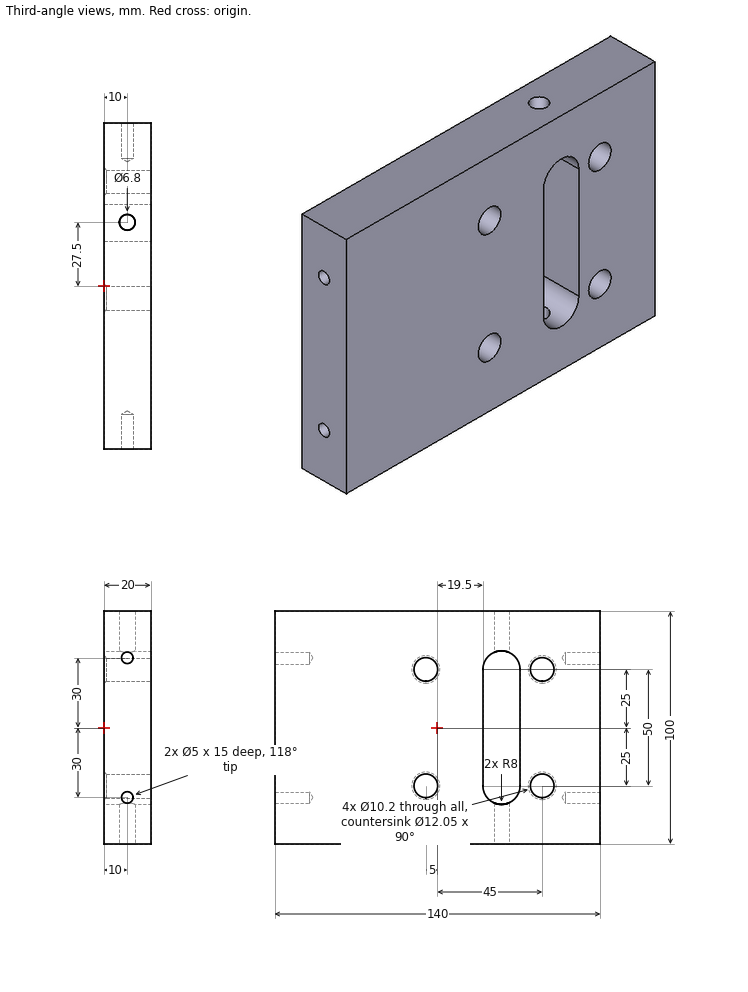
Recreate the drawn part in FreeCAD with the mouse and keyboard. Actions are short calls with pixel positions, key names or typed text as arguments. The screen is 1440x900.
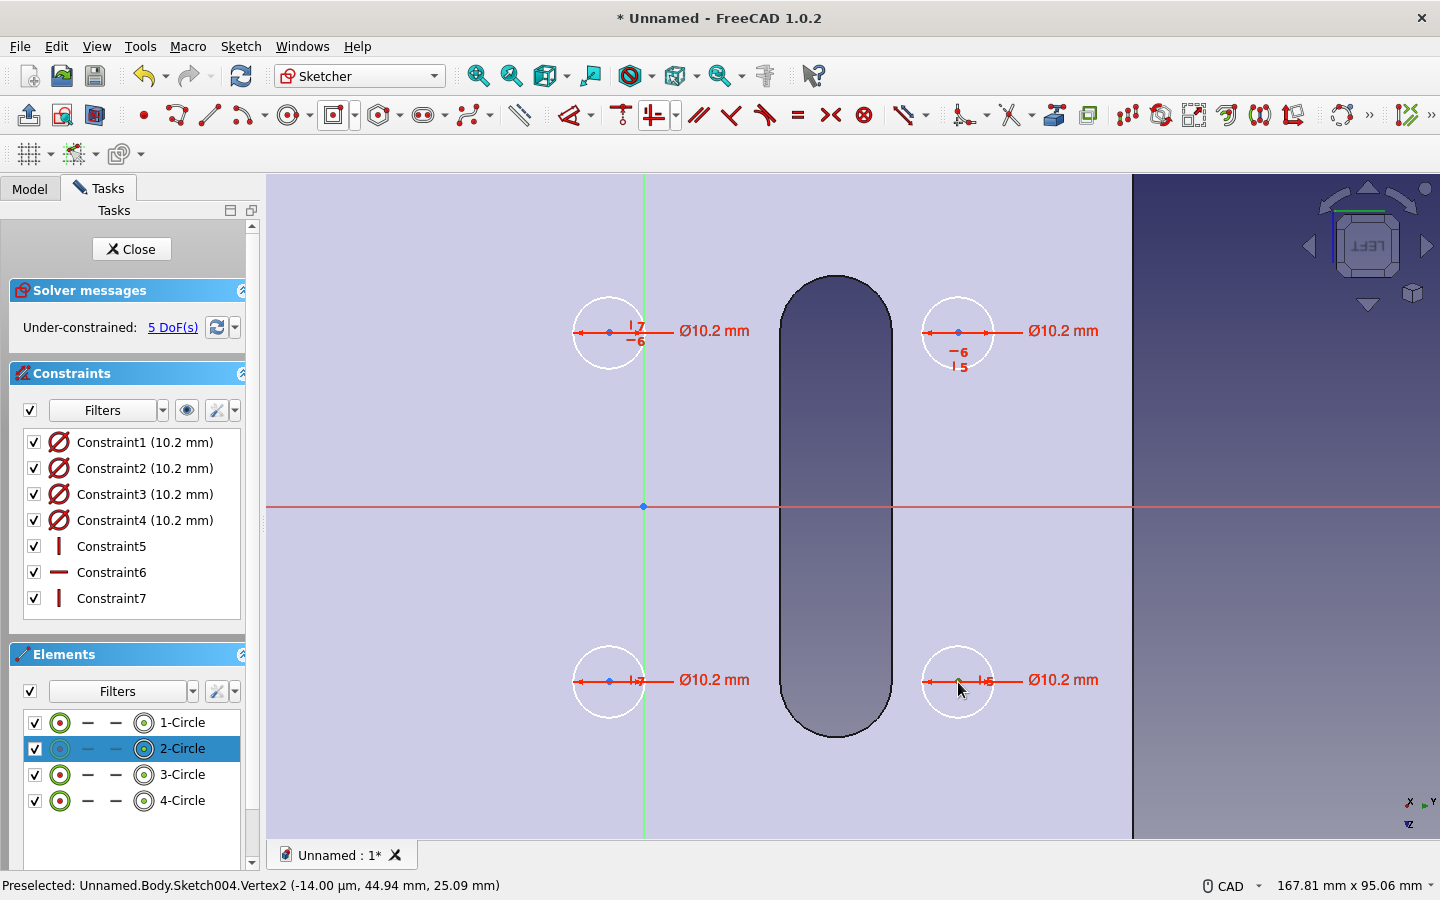
click(609, 682)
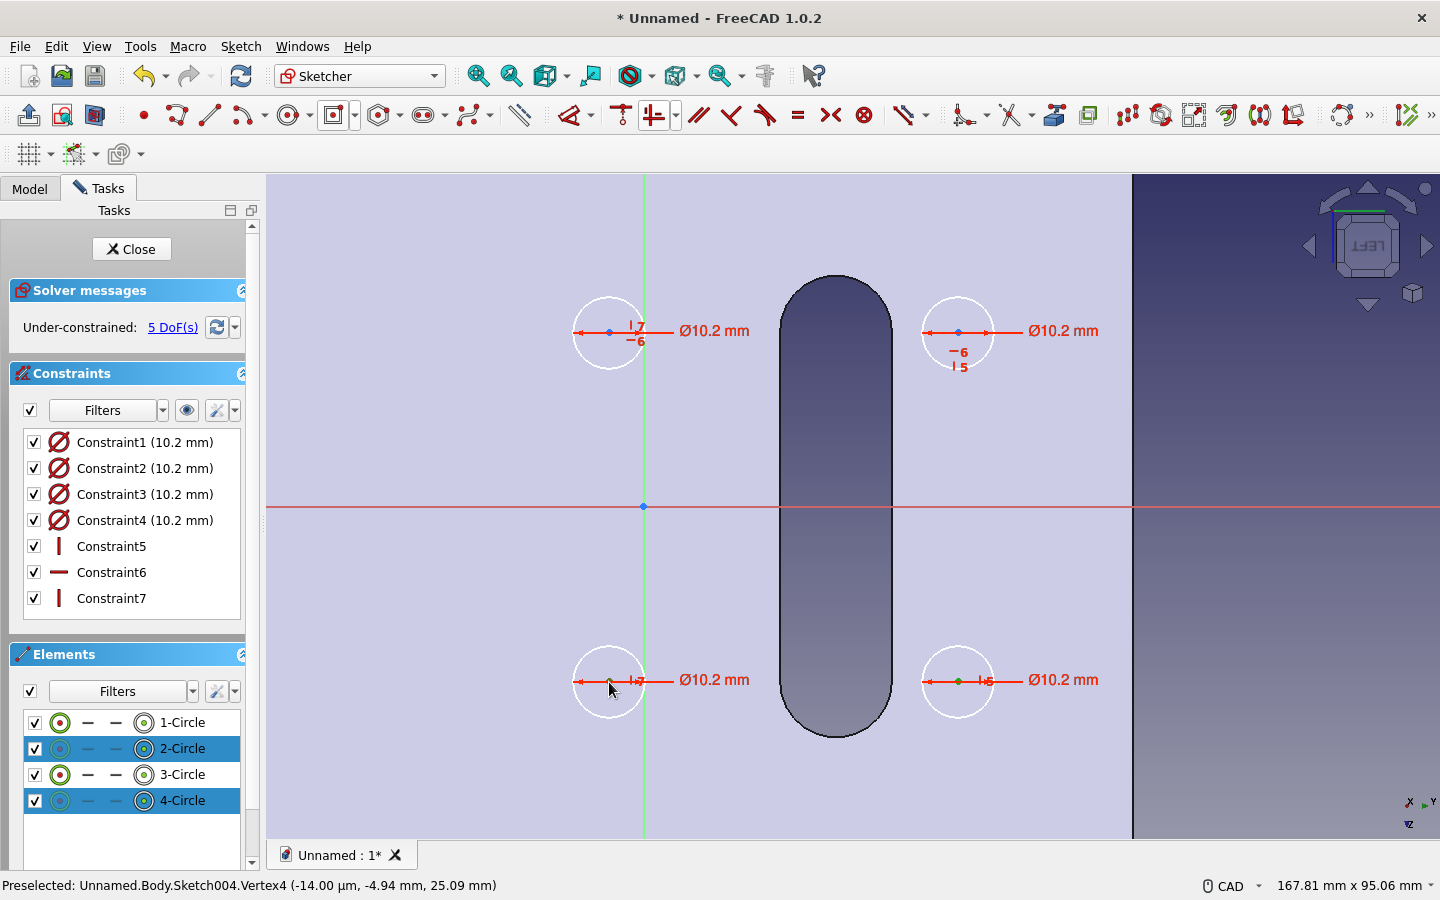
click(676, 116)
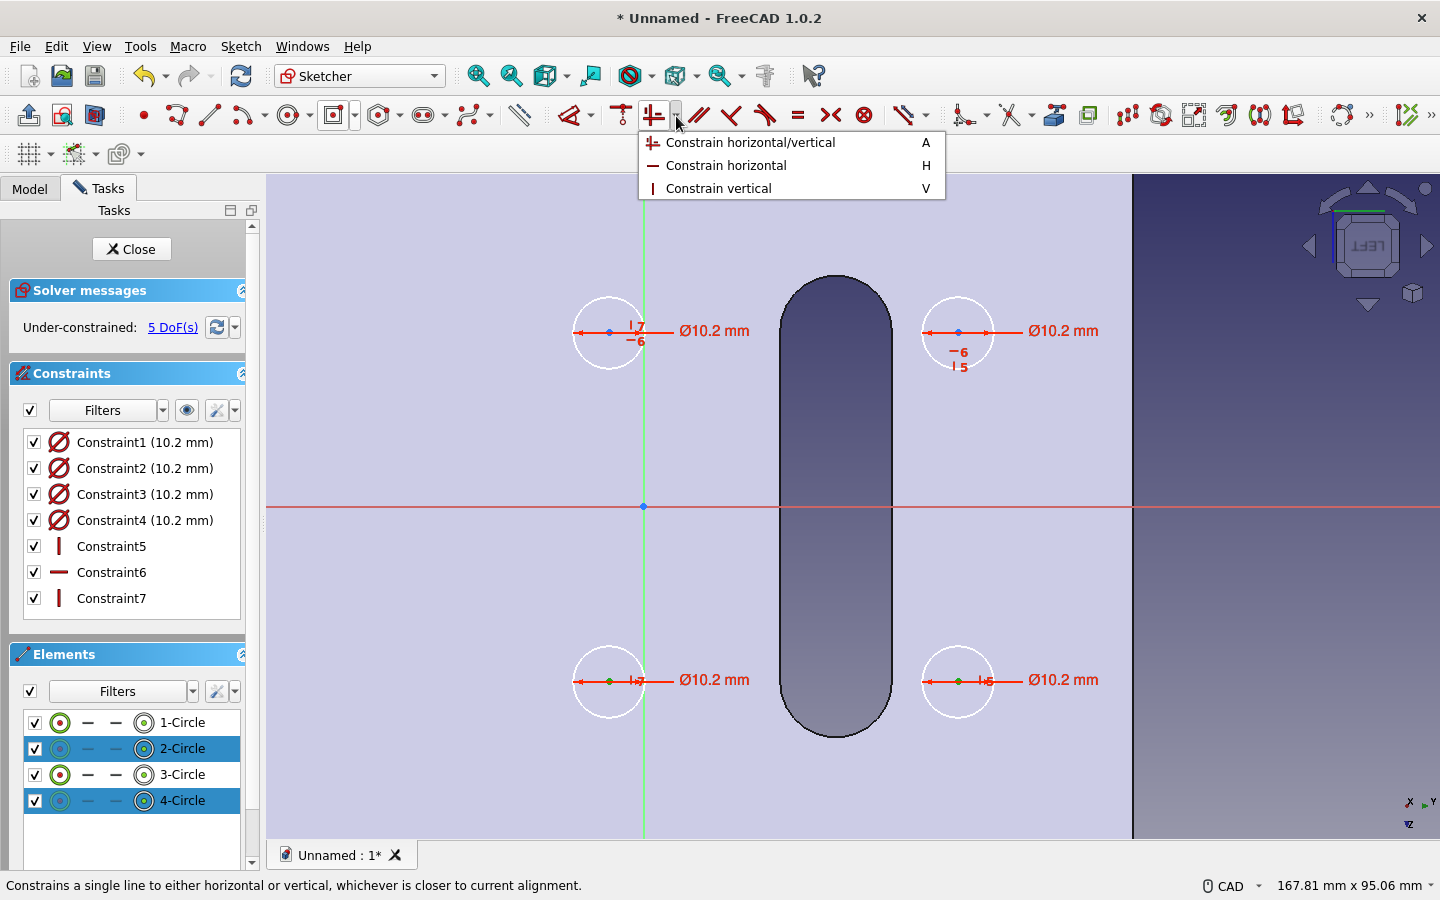
click(792, 166)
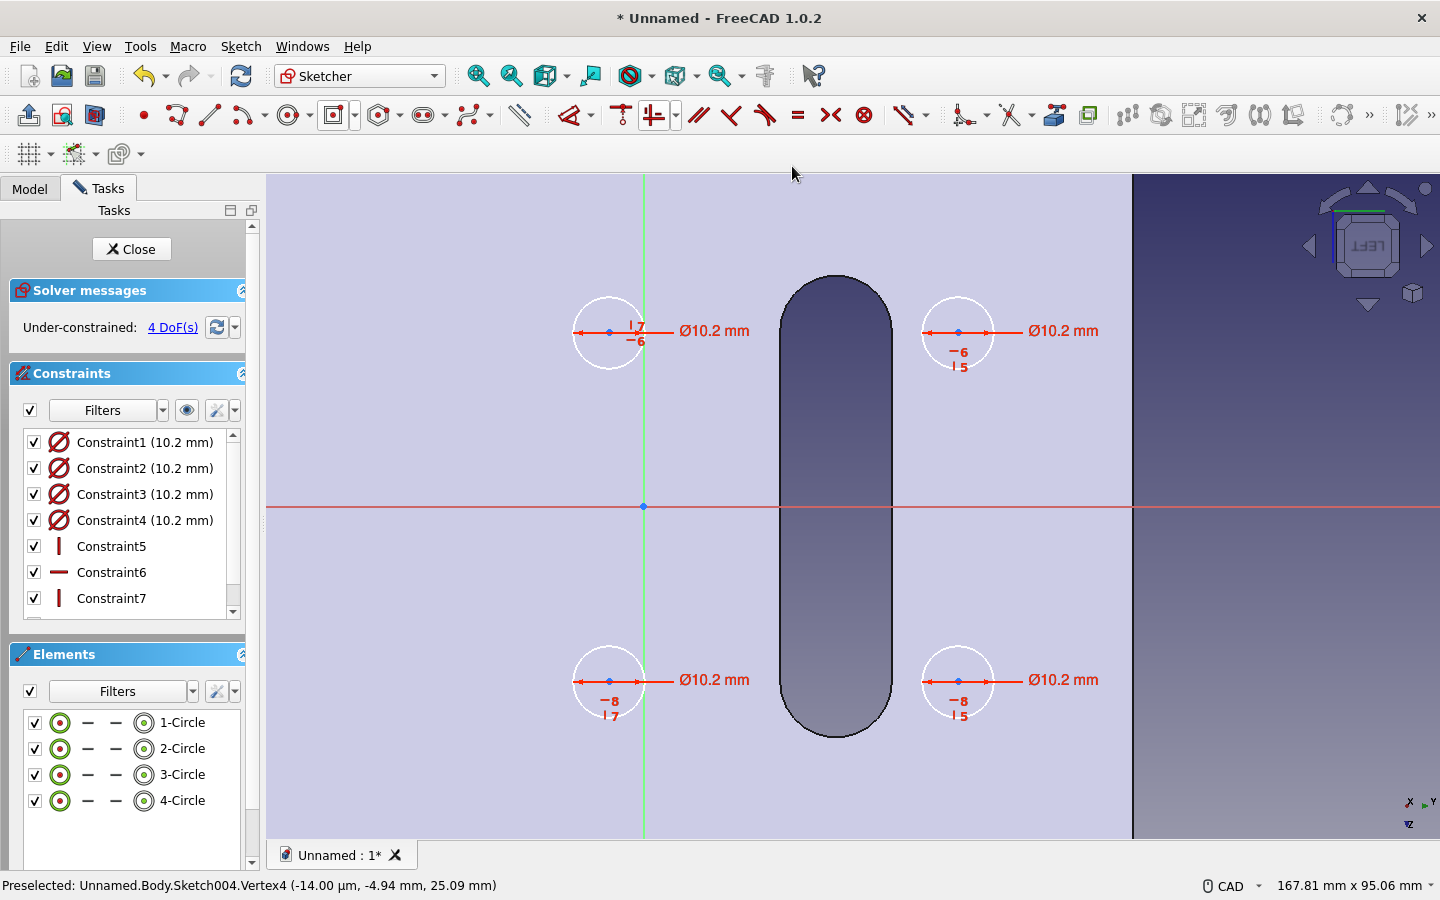
click(568, 116)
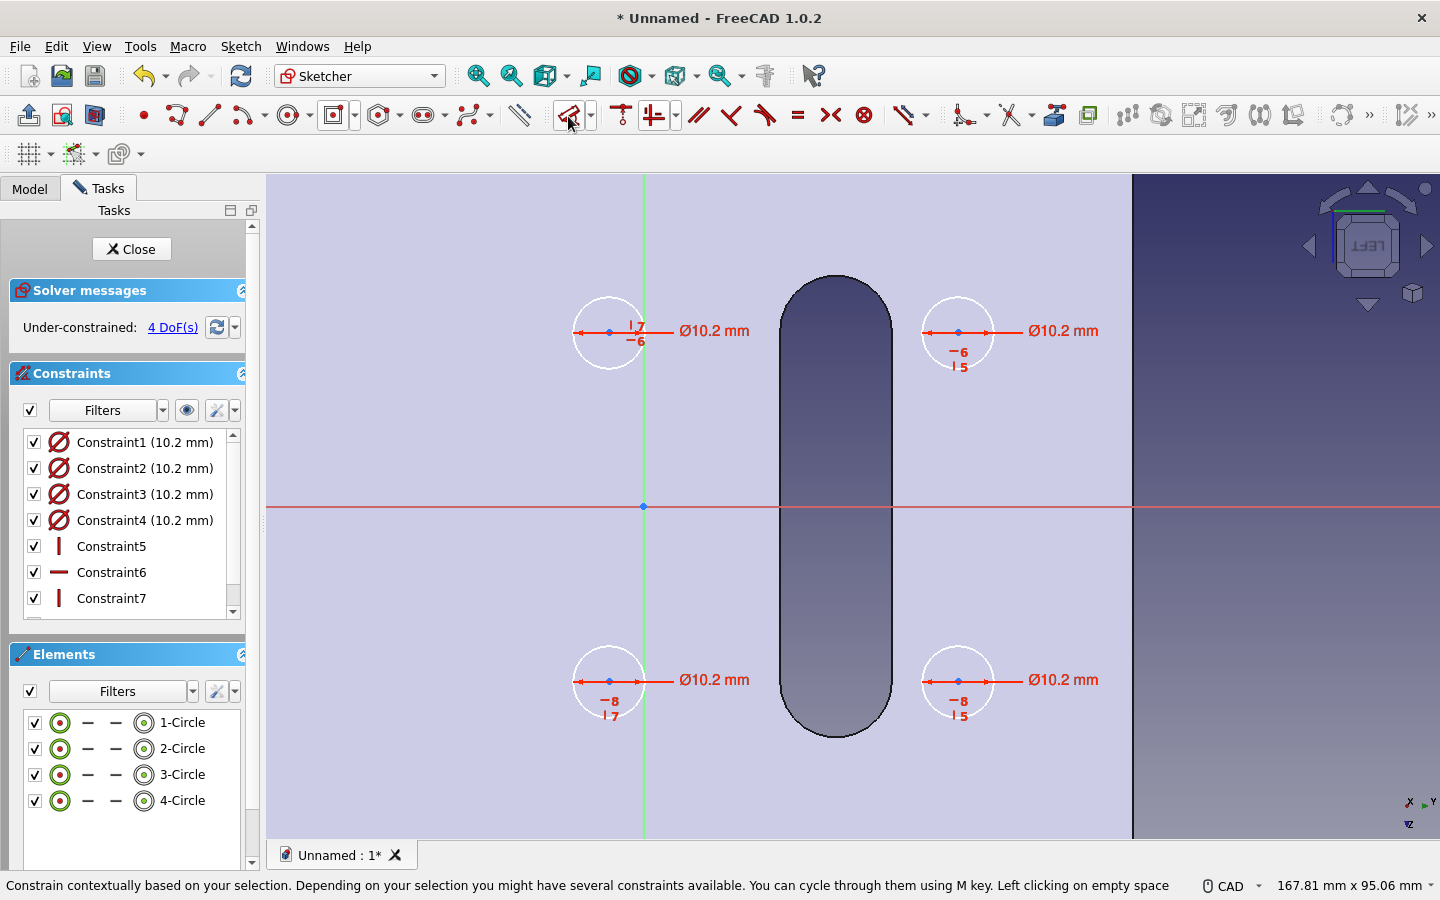
click(609, 333)
click(626, 540)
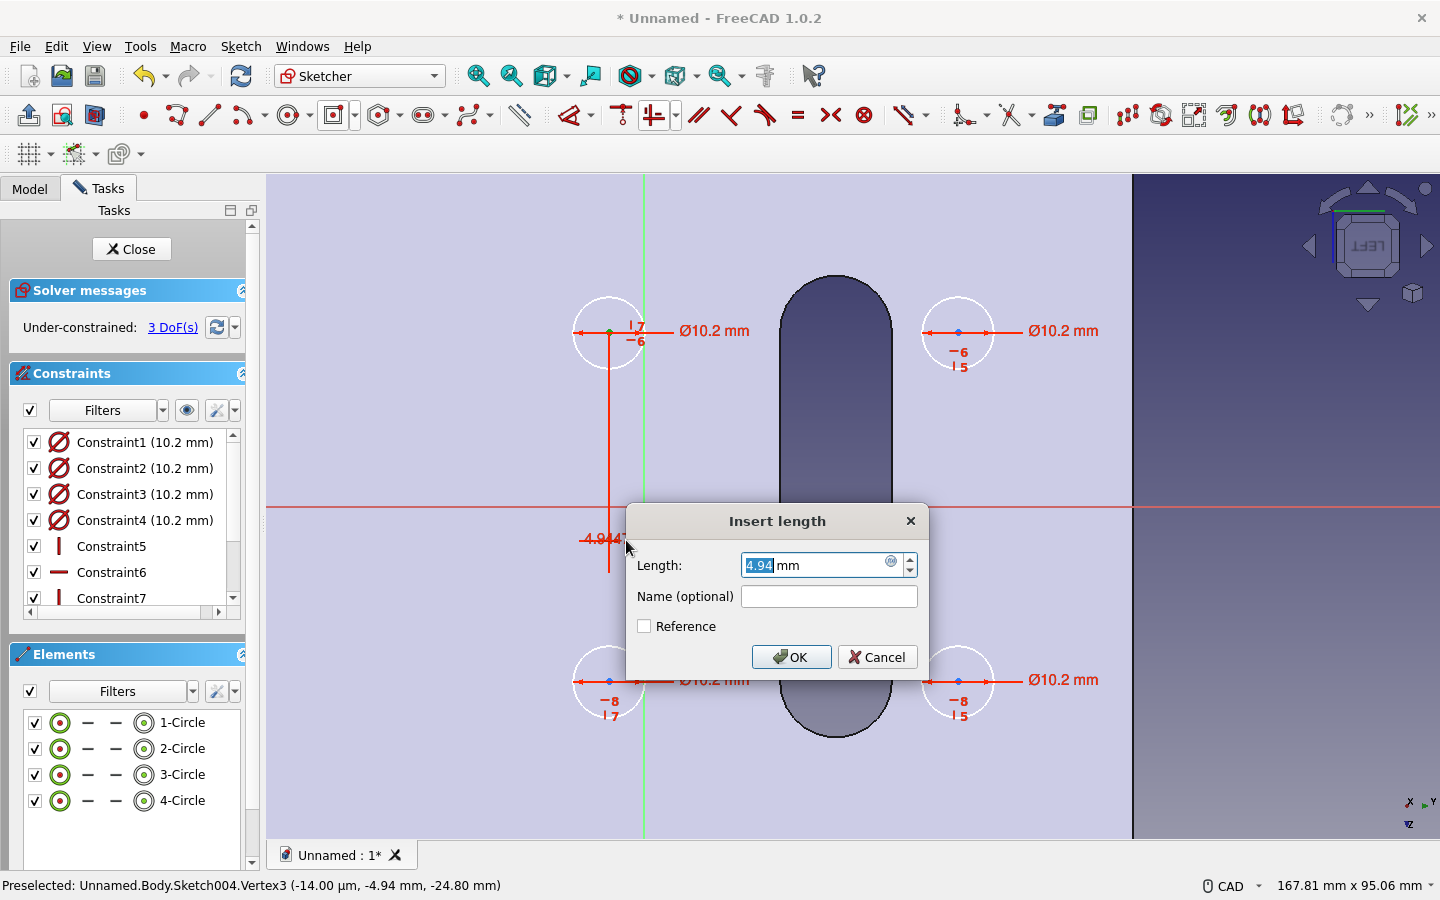
text(5)
key(Return)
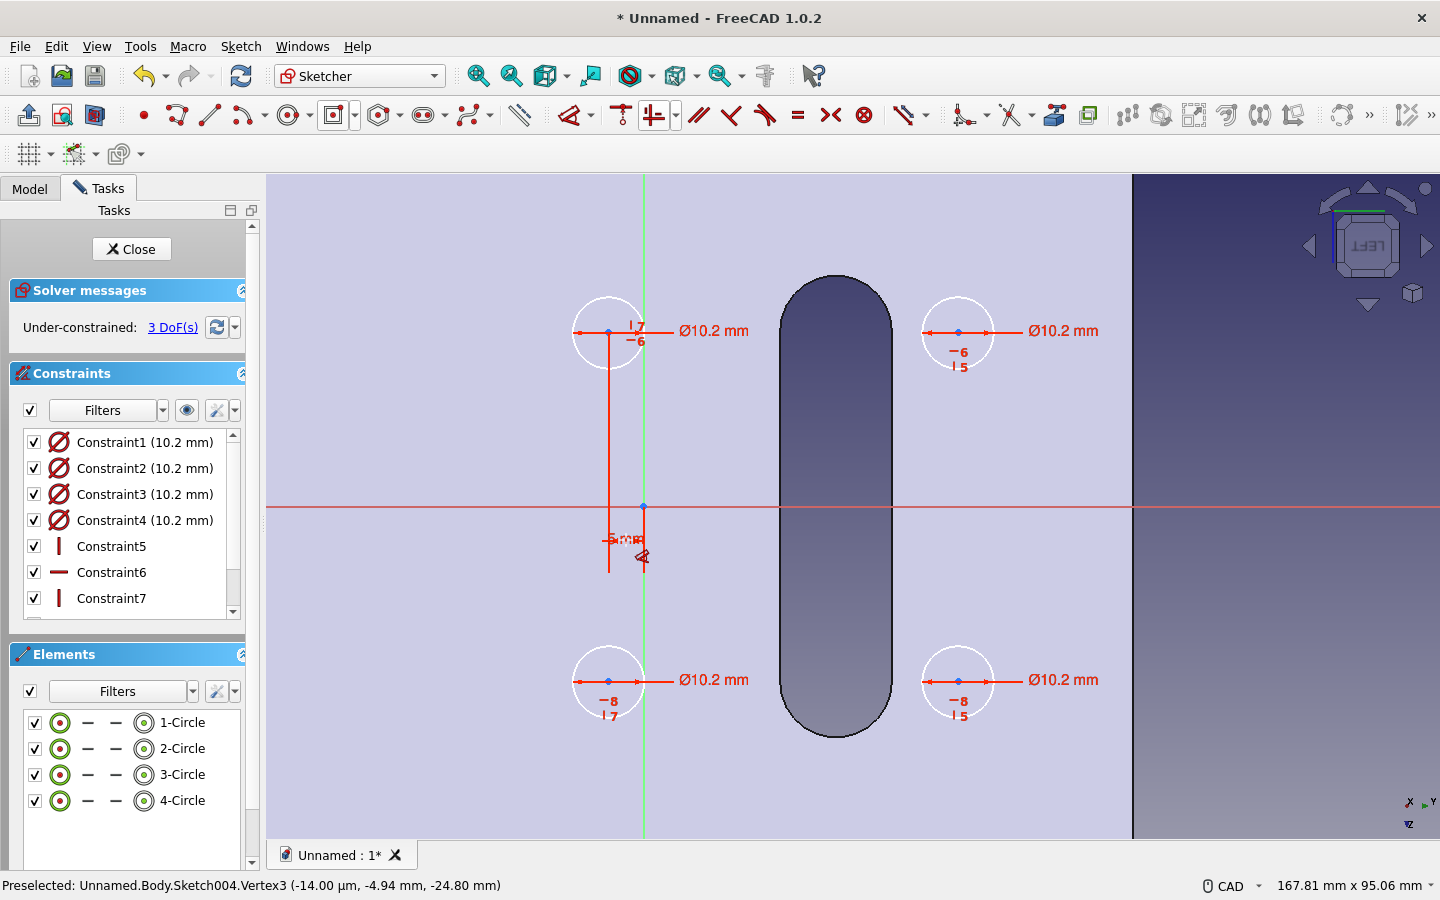
click(958, 333)
click(801, 299)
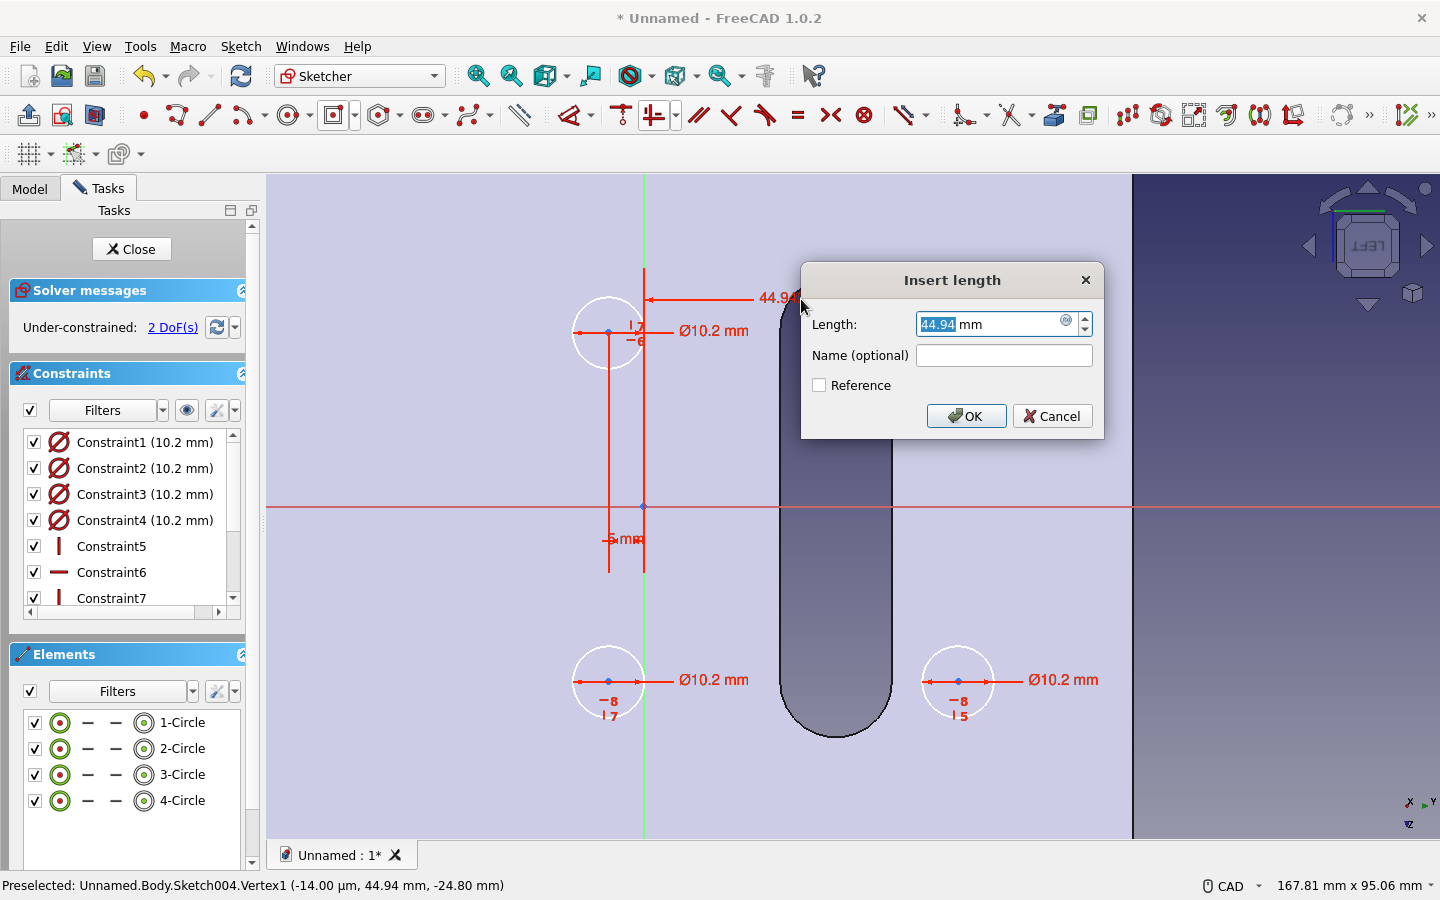
text(45)
key(Return)